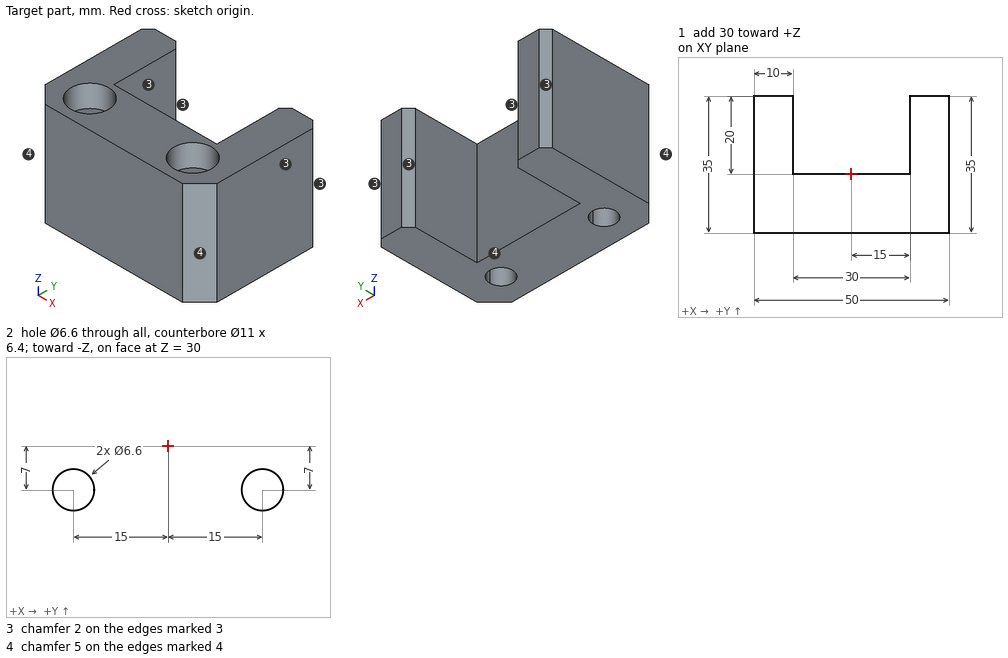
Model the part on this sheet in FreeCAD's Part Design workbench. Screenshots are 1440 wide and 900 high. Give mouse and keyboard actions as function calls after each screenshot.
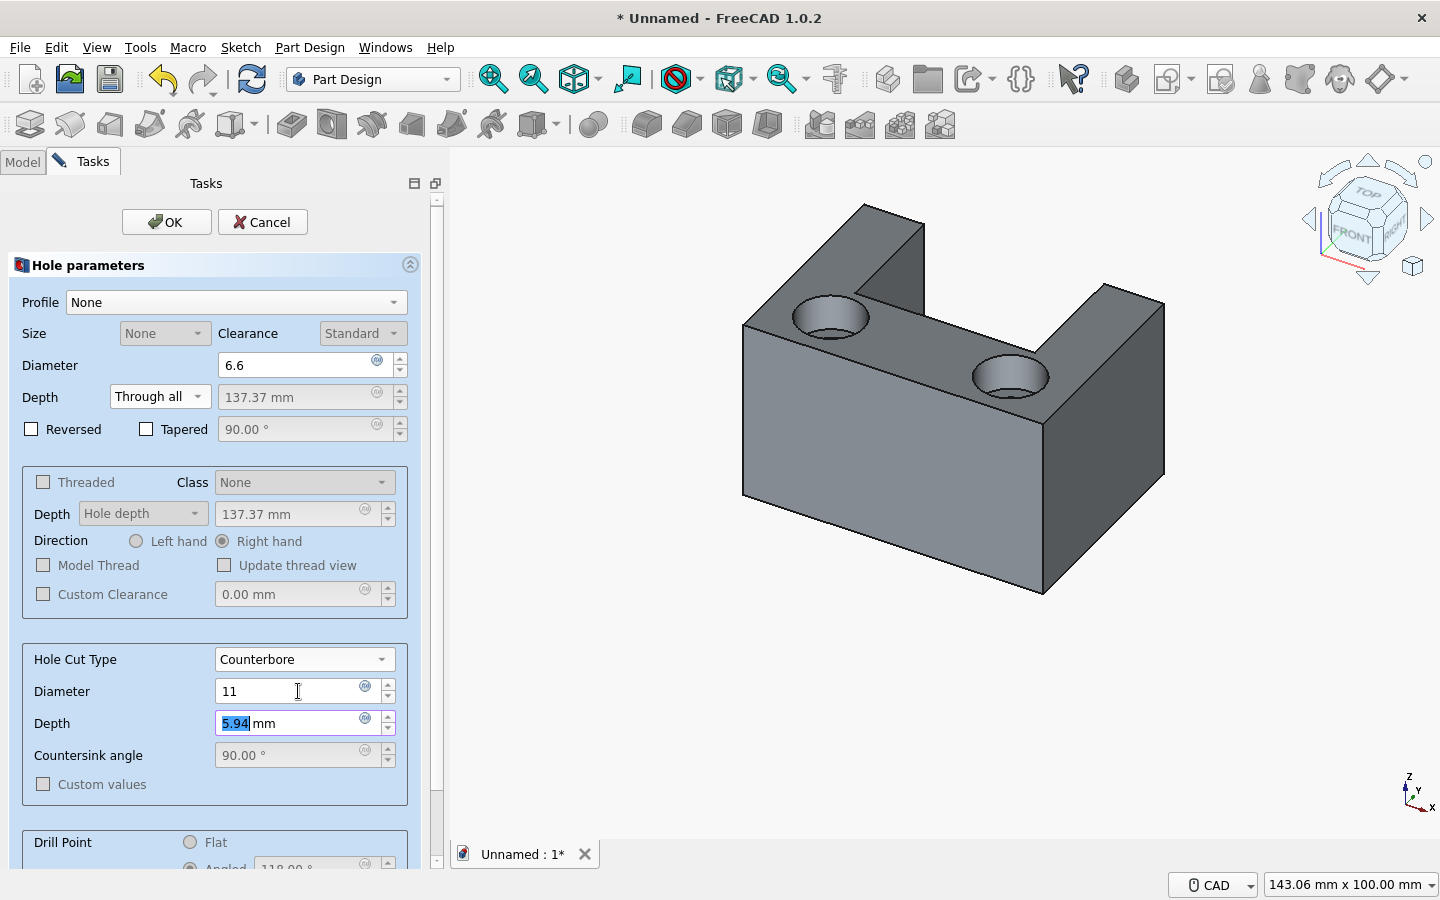
text(6.4)
key(Tab)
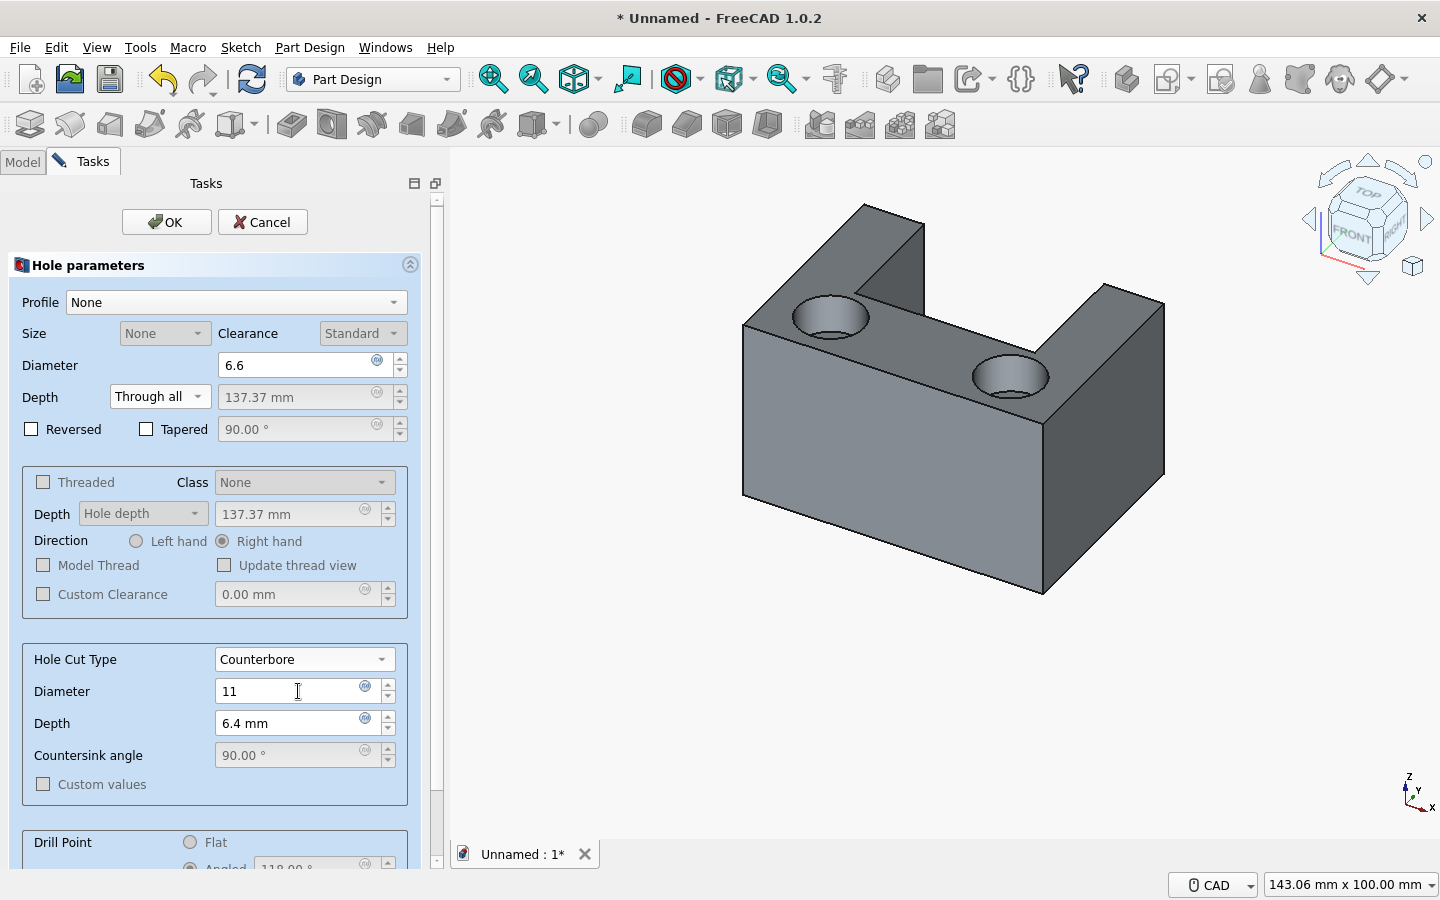
click(167, 222)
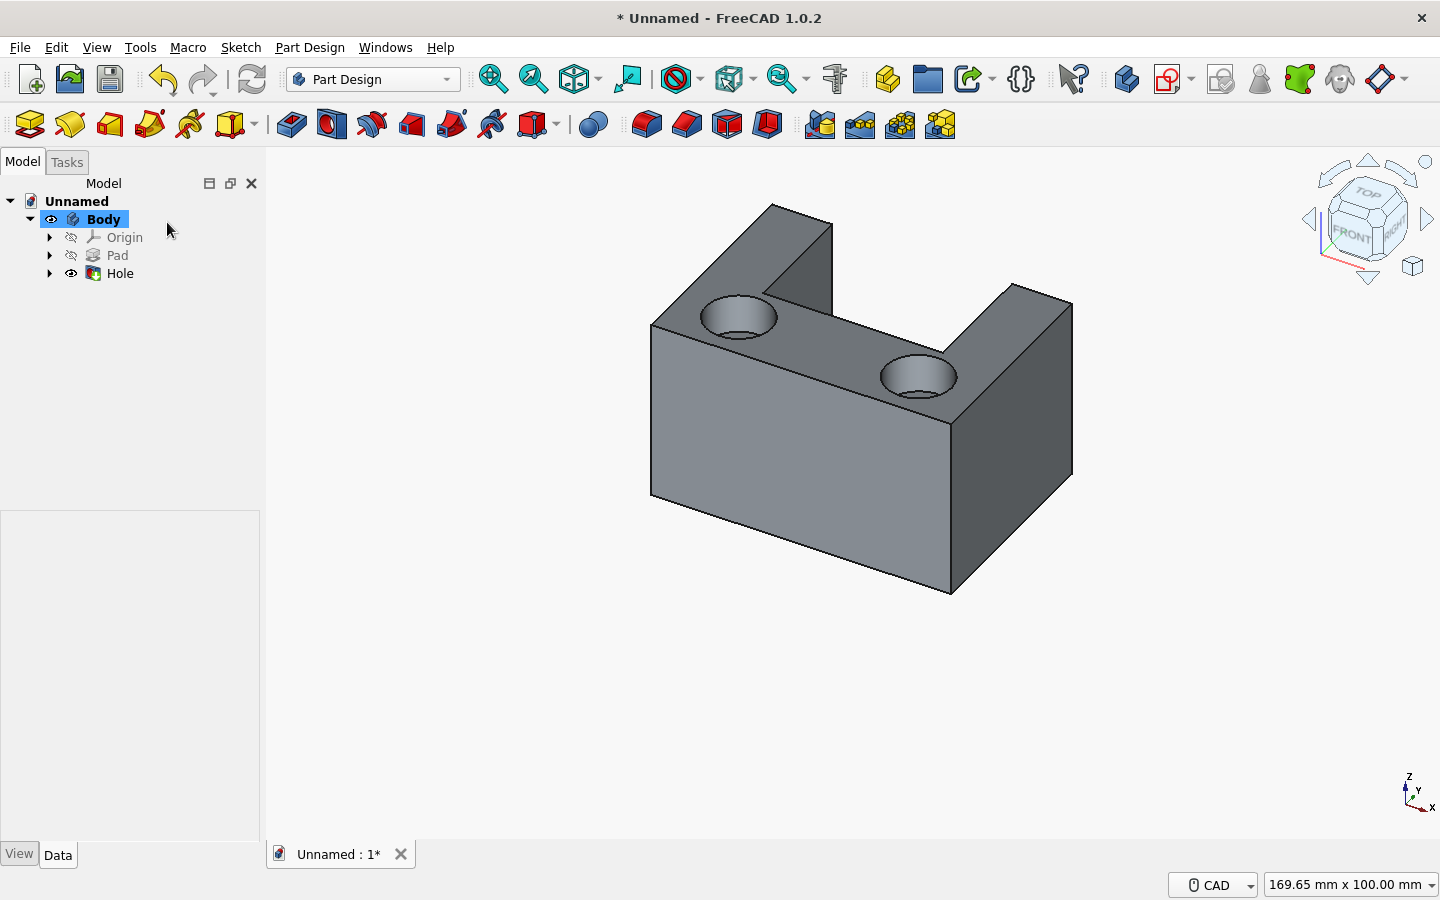
key(0)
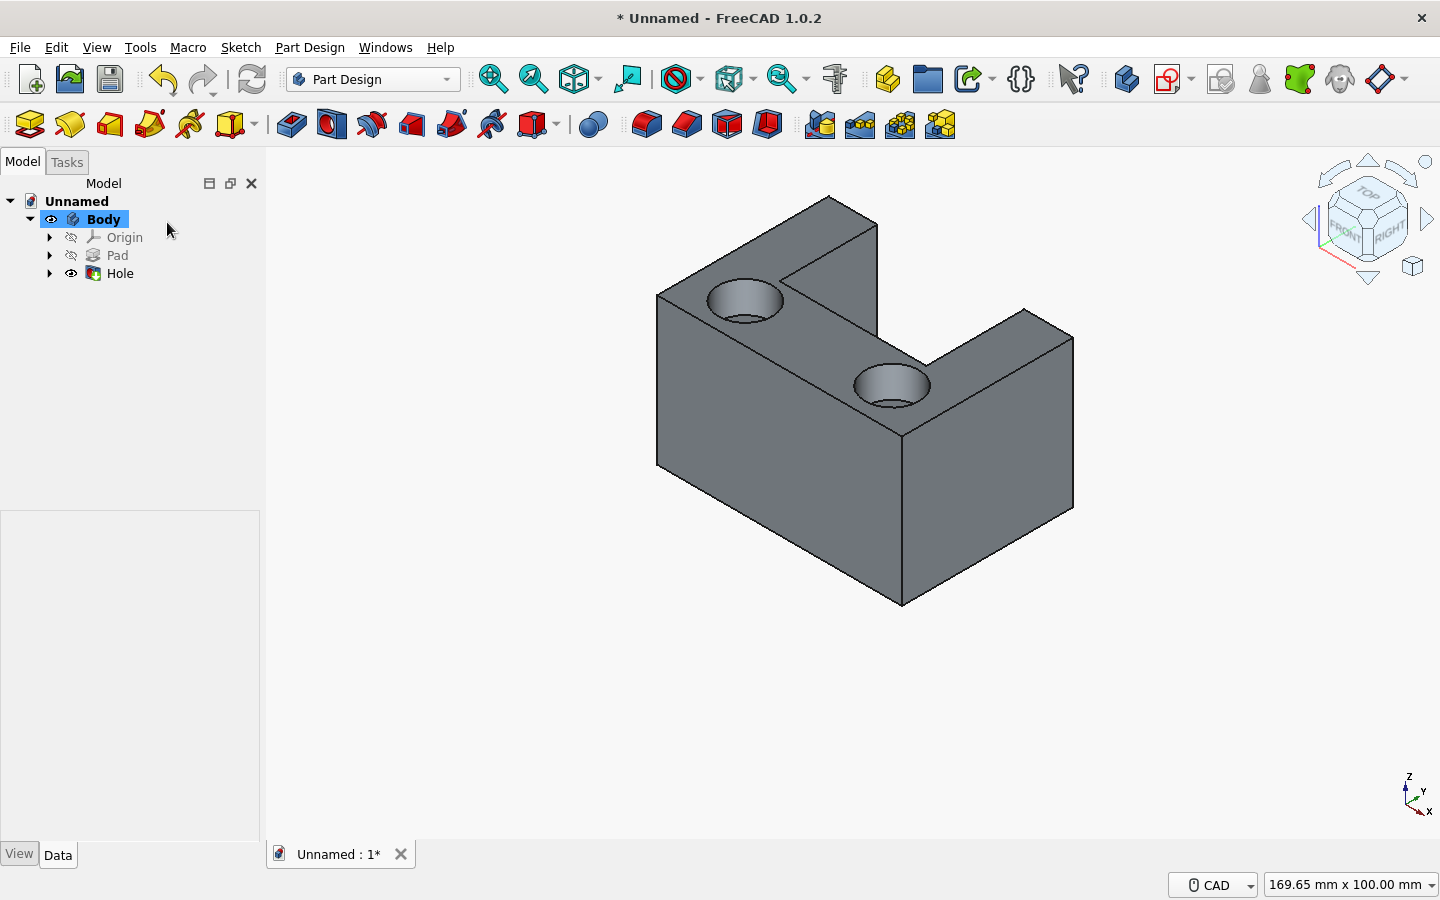
key(2)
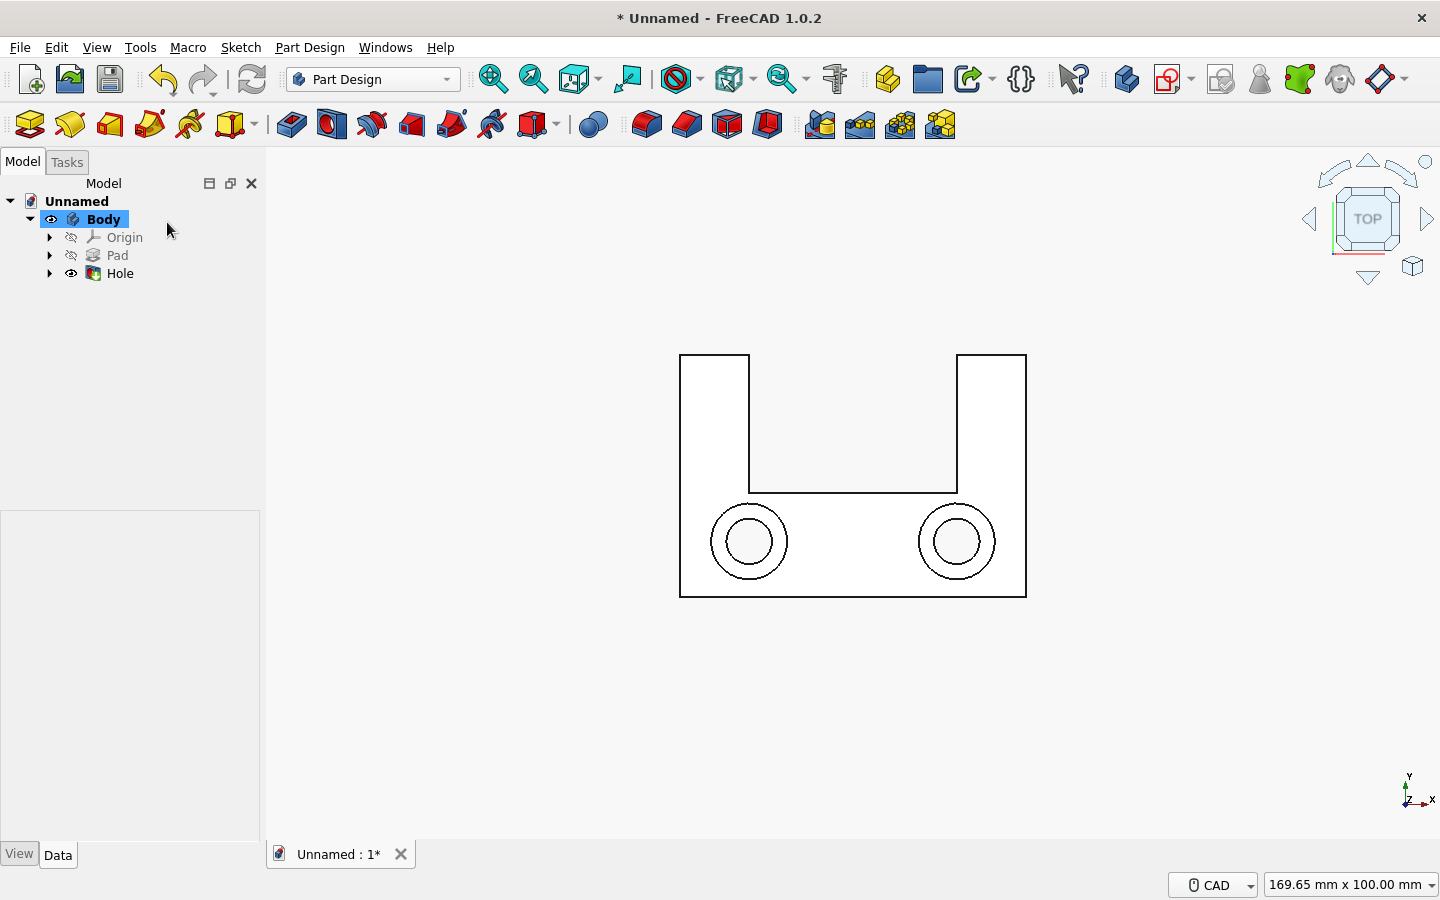
click(494, 80)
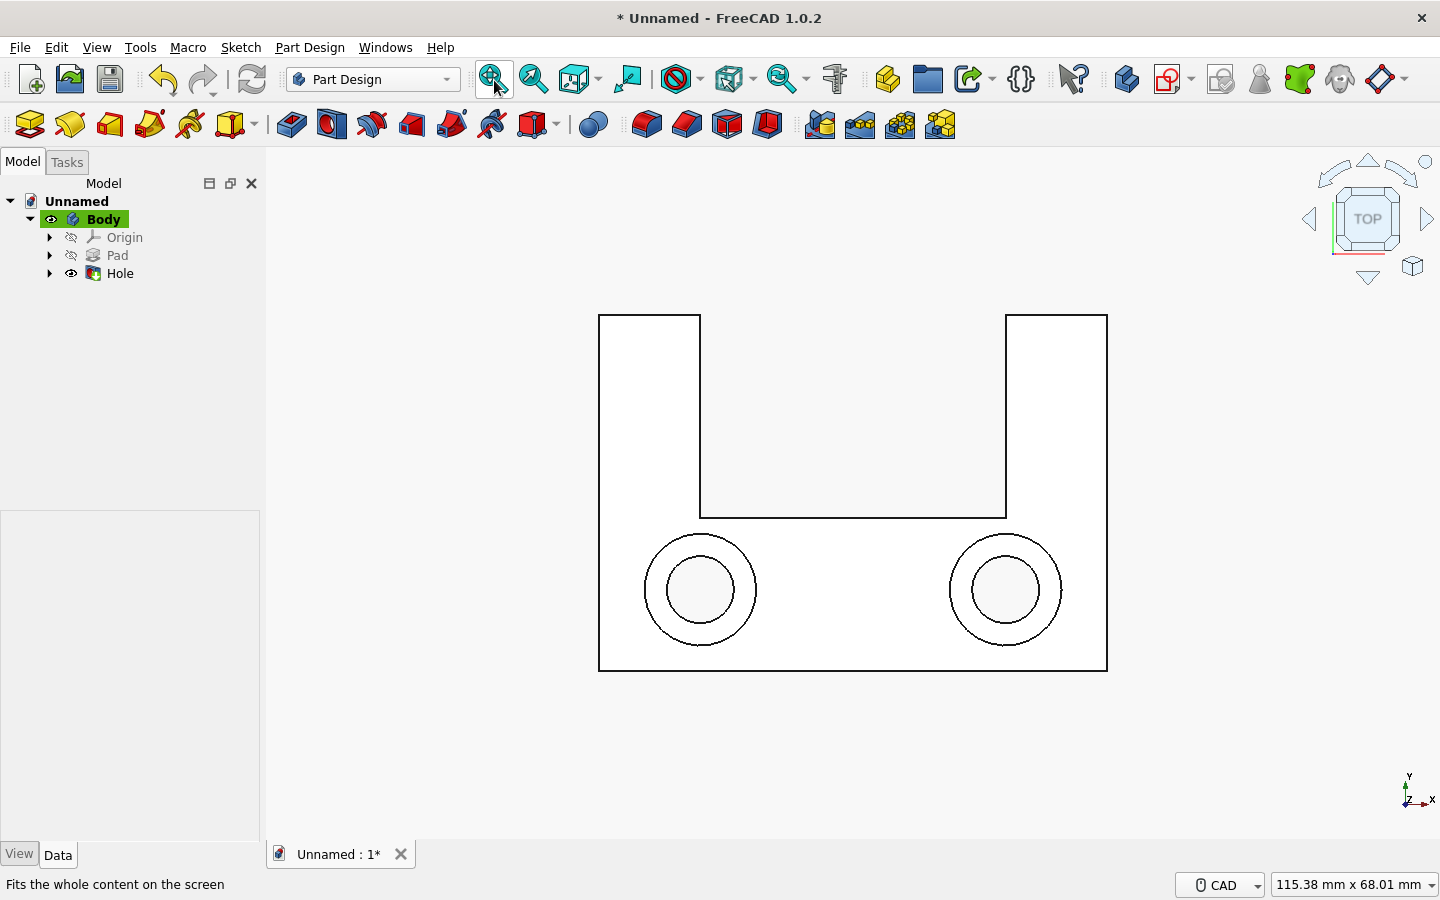
key(1)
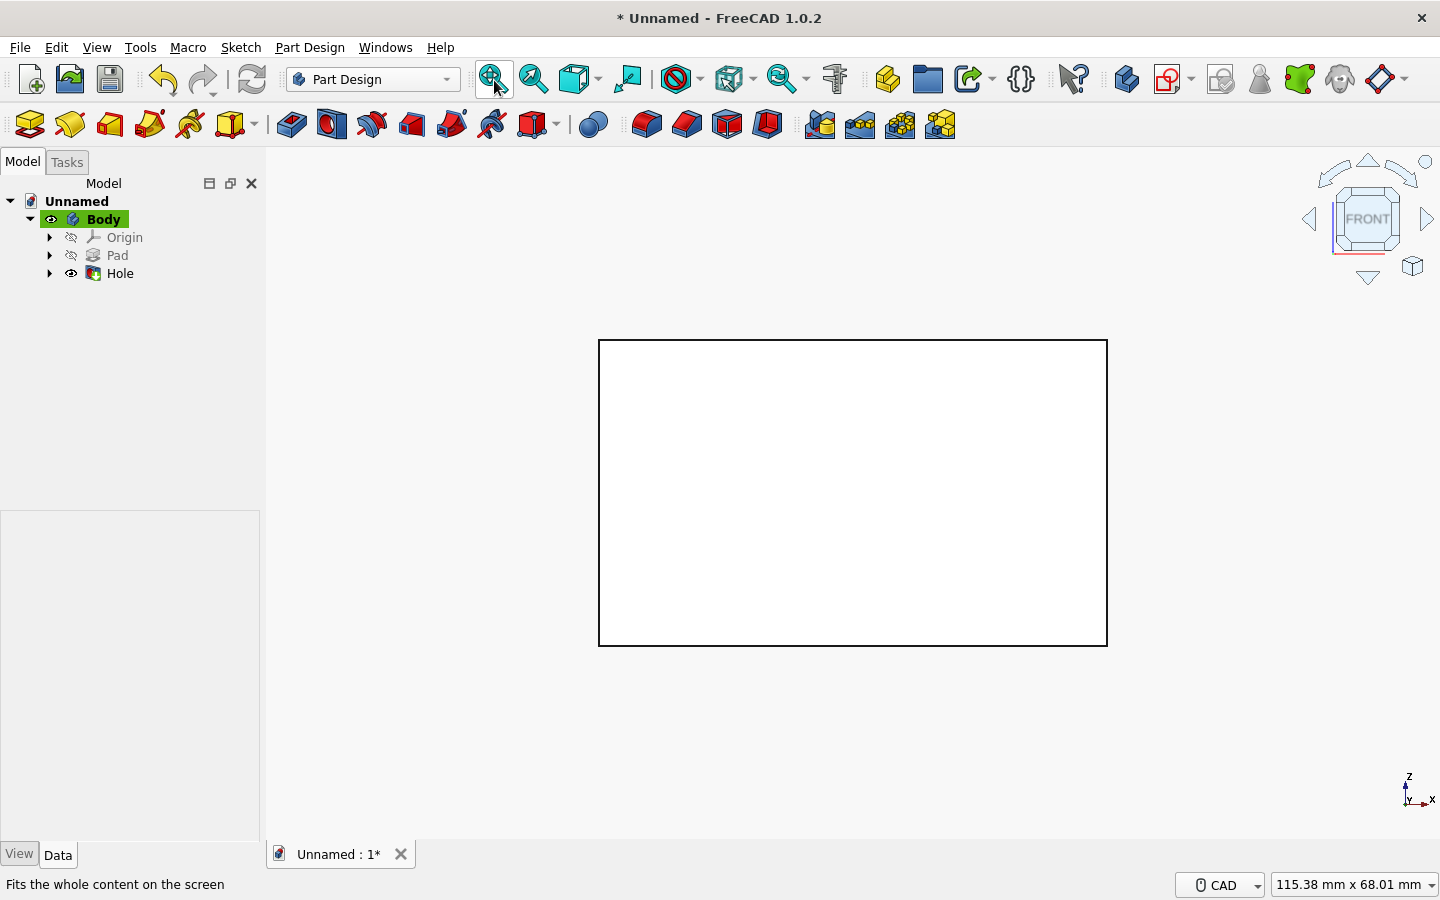
click(494, 80)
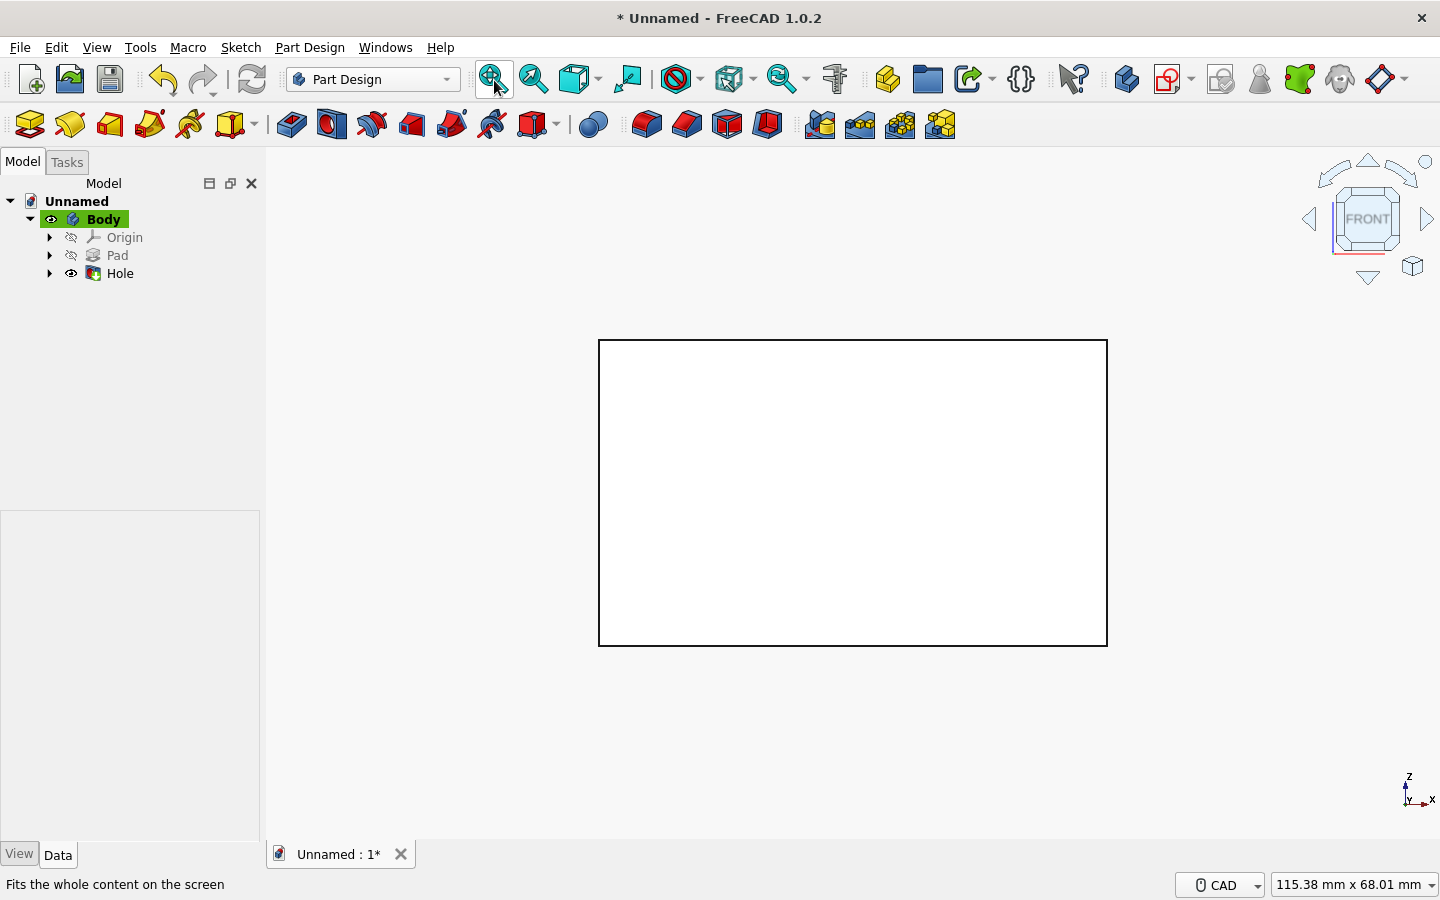
key(3)